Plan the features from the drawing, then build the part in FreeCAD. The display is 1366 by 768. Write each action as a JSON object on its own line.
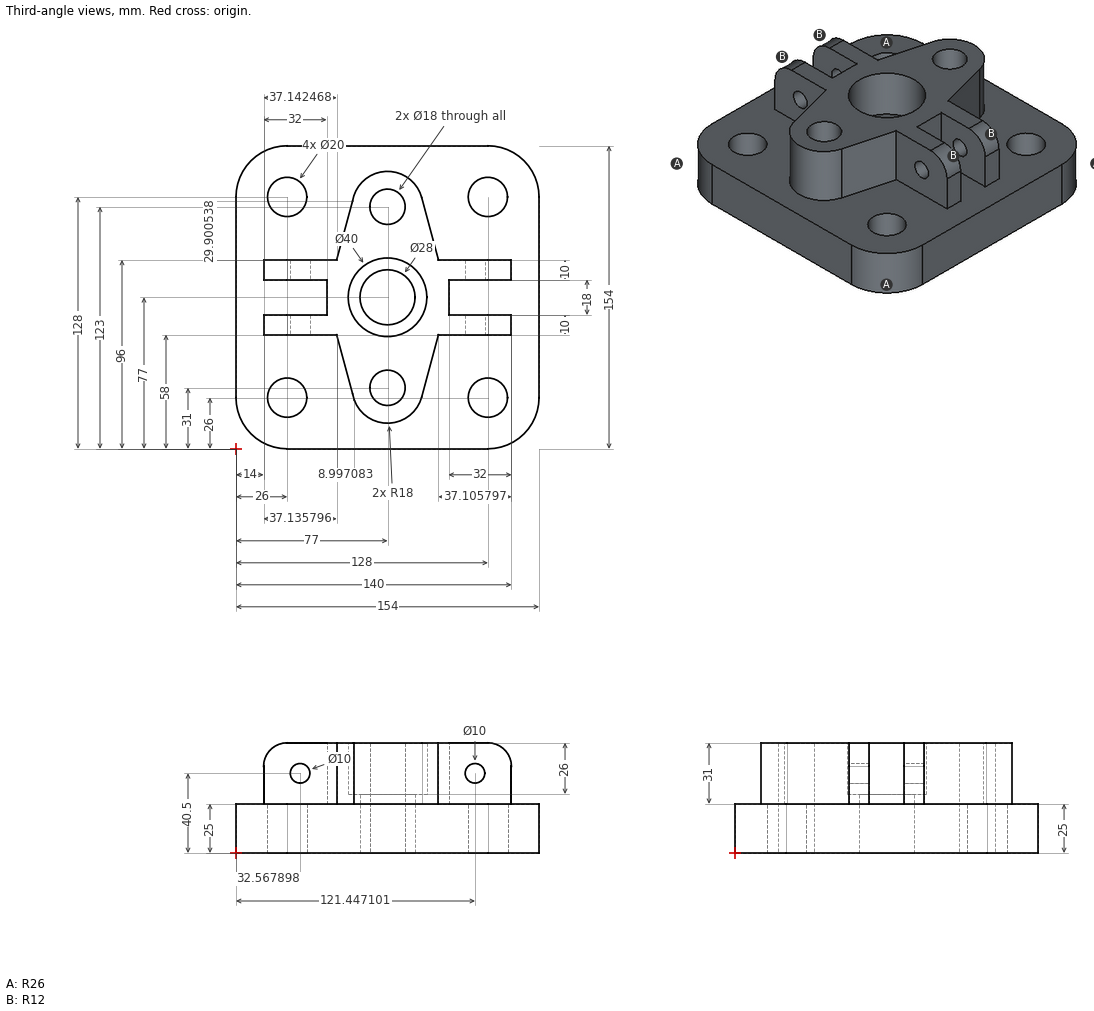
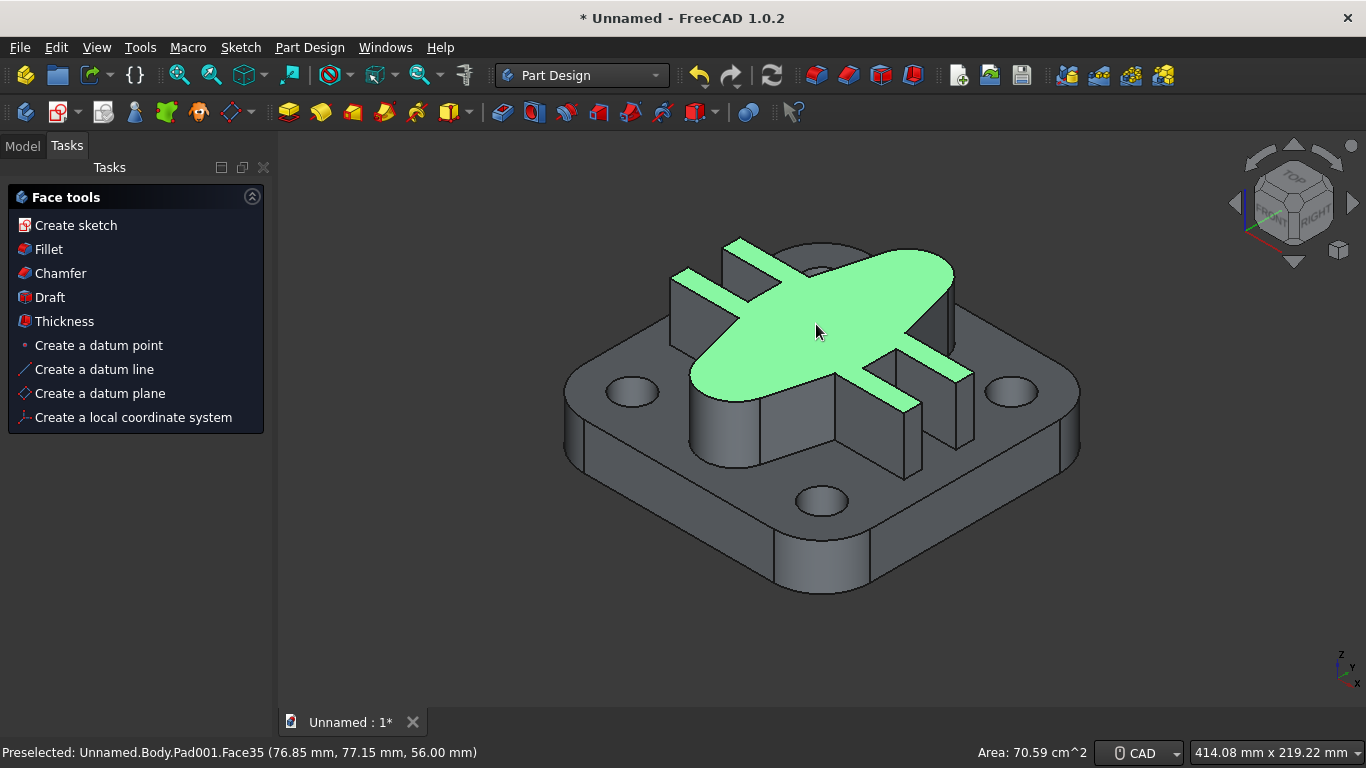
{"action": "left_click", "coordinate": [58, 112]}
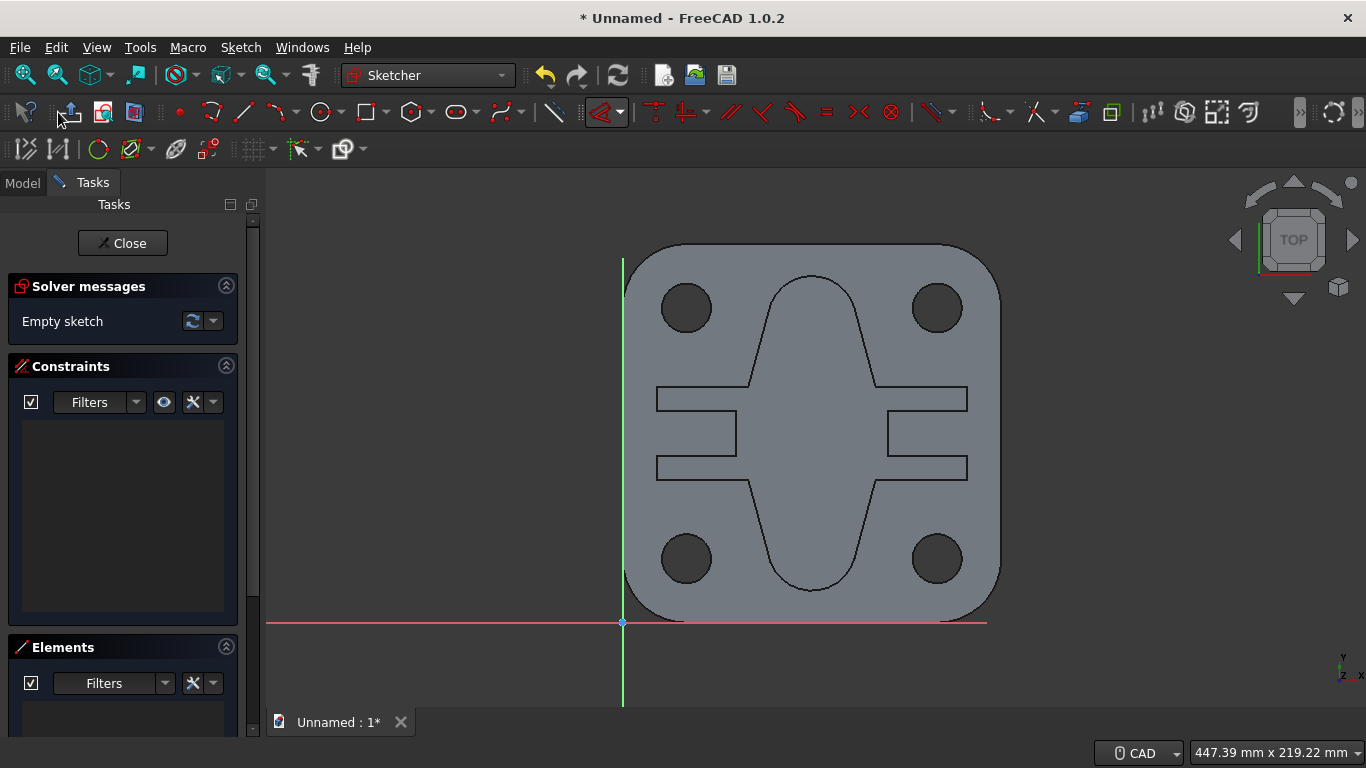
{"action": "left_click", "coordinate": [322, 112]}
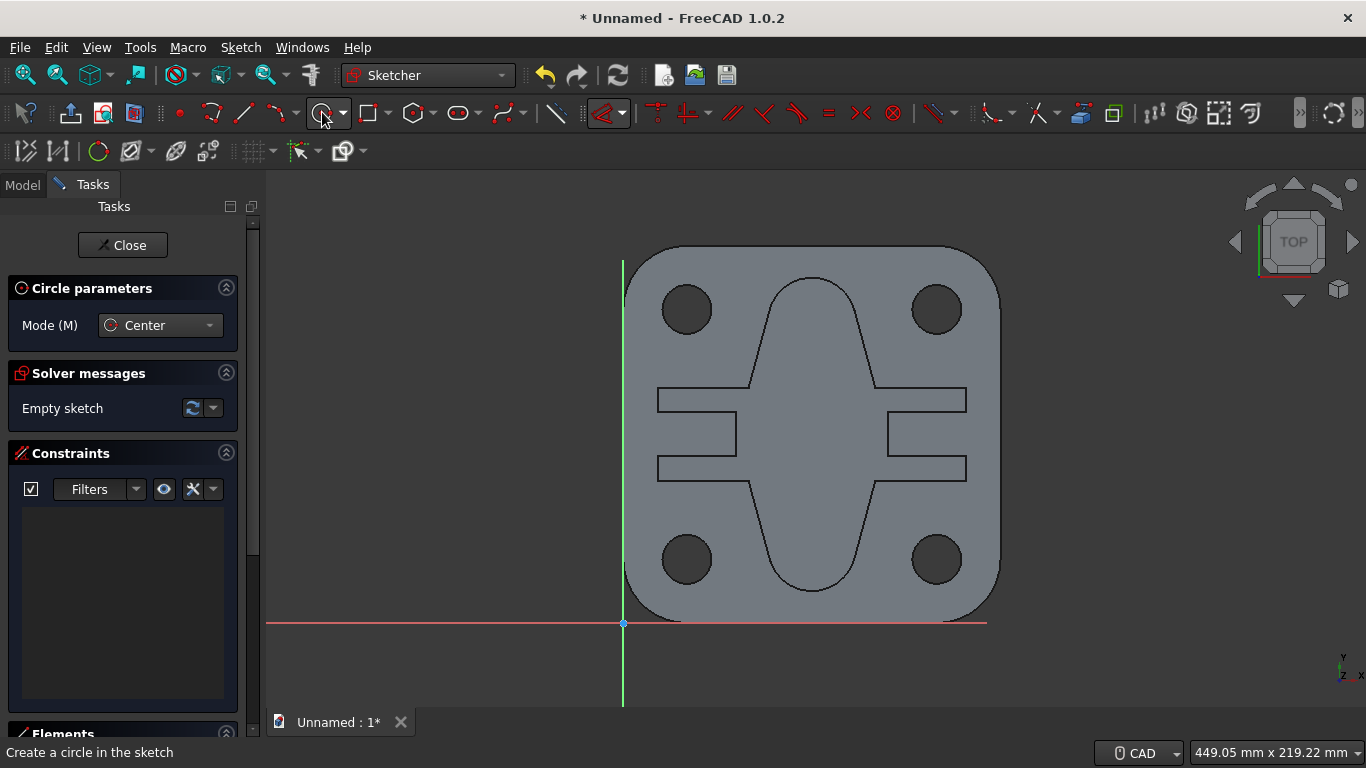
{"action": "left_click", "coordinate": [812, 322]}
{"action": "left_click", "coordinate": [827, 306]}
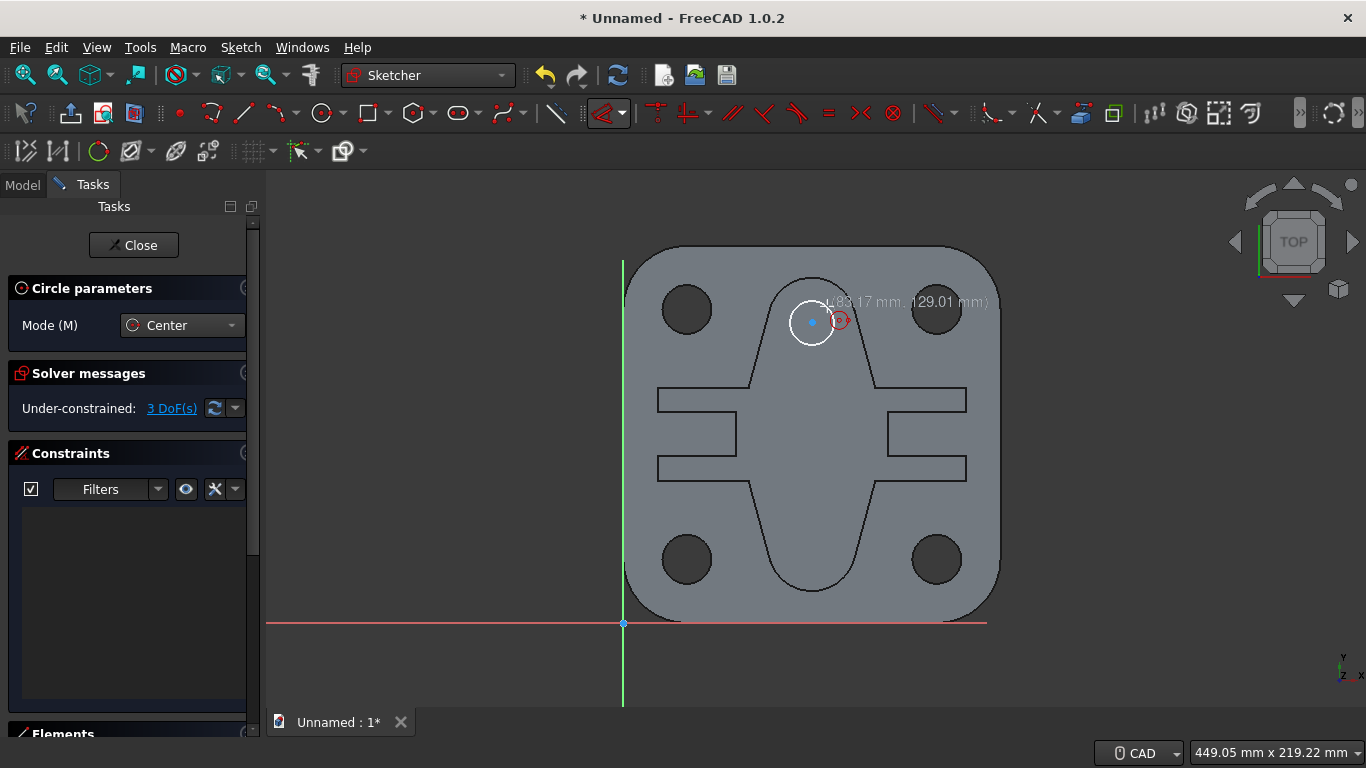
{"action": "left_click", "coordinate": [812, 547]}
{"action": "left_click", "coordinate": [827, 531]}
{"action": "key", "text": "Escape"}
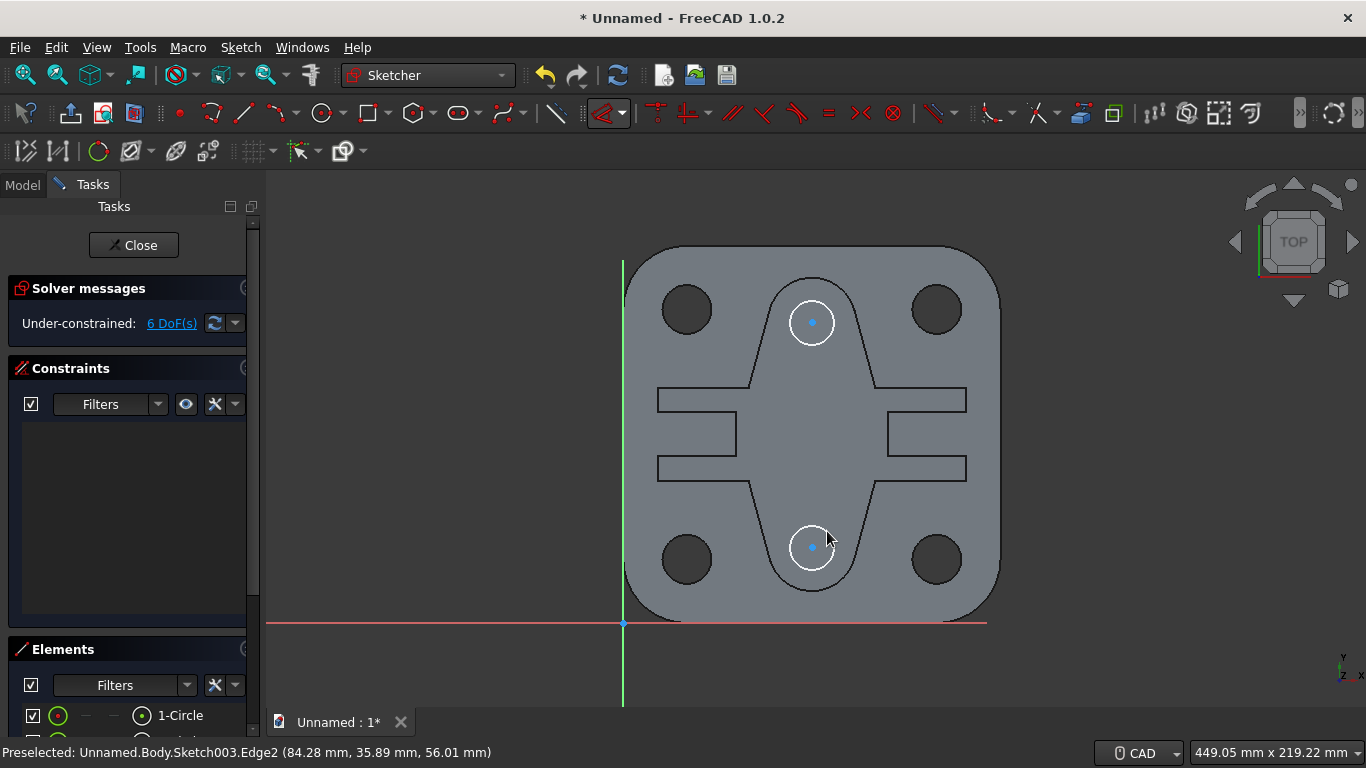
{"action": "left_click", "coordinate": [827, 307]}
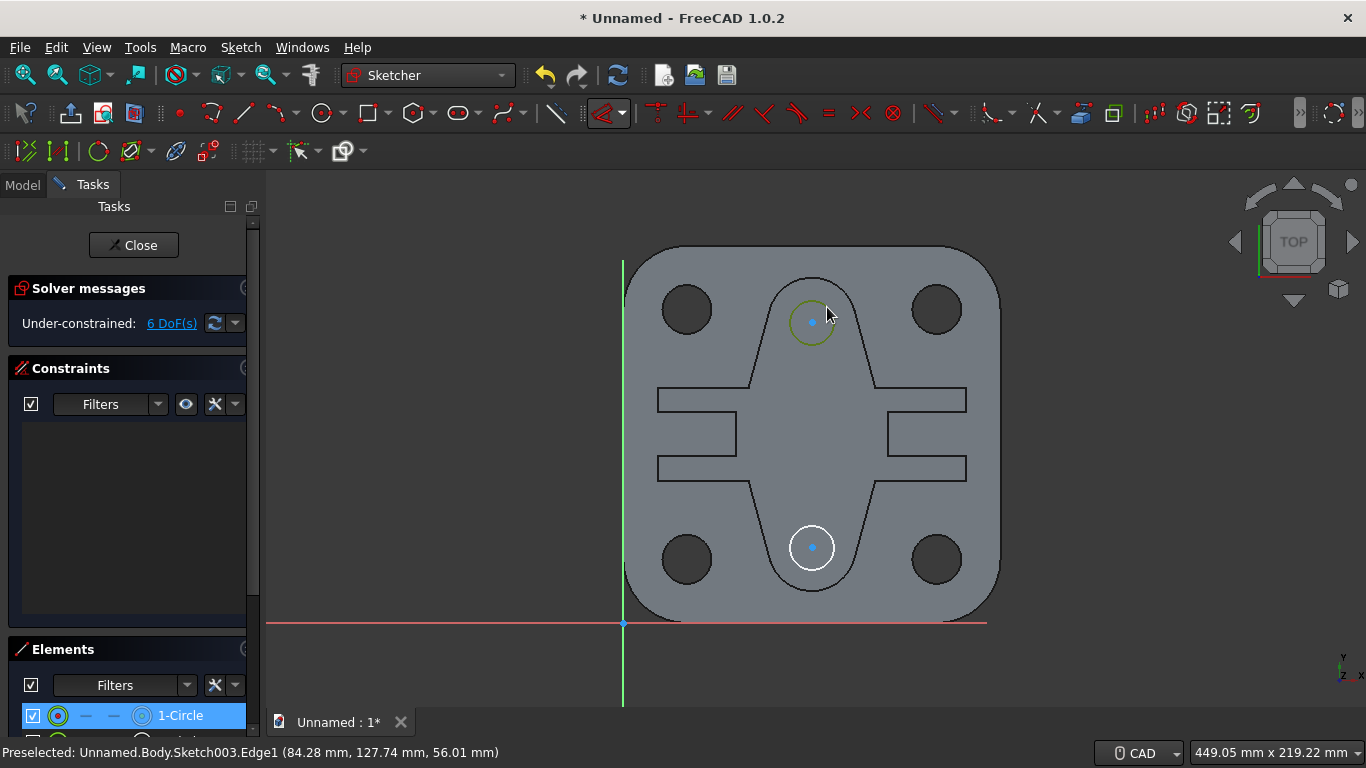
{"action": "left_click", "coordinate": [827, 532]}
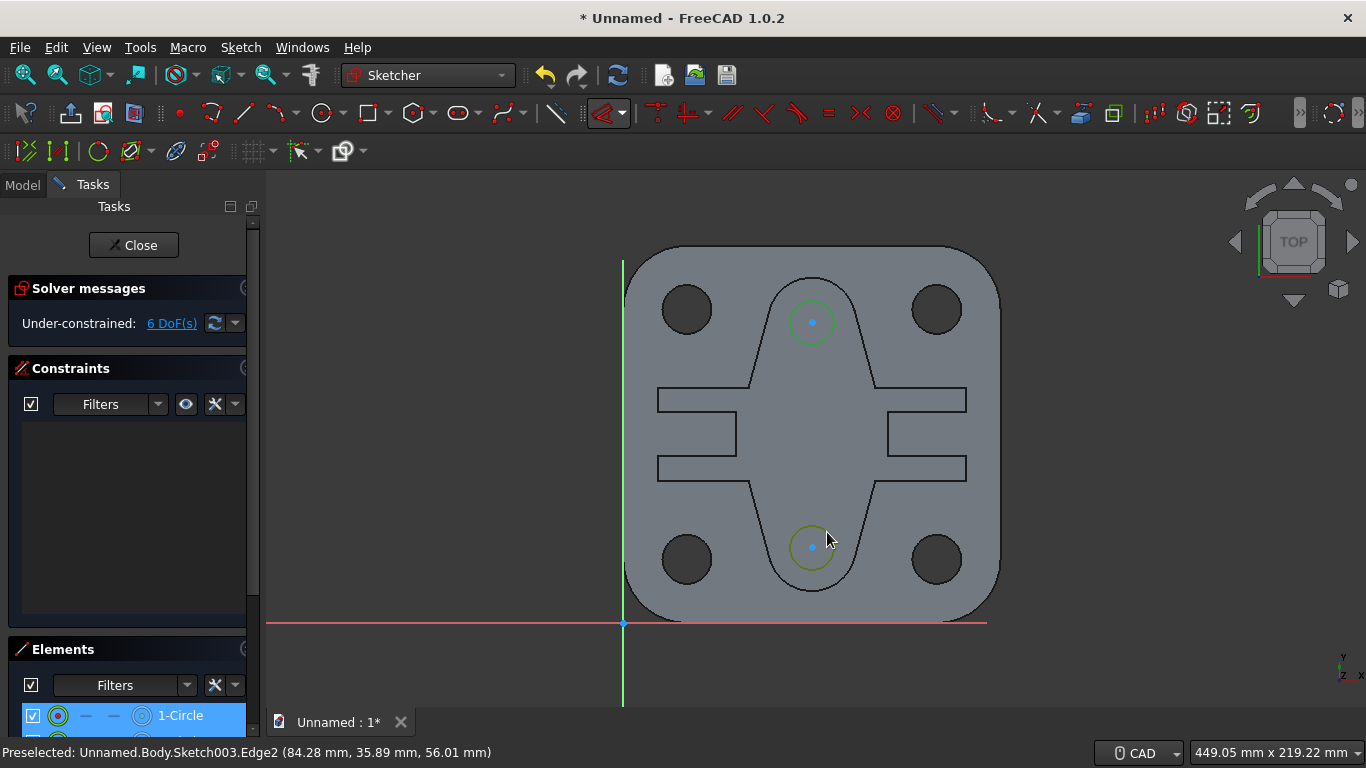
{"action": "left_click", "coordinate": [830, 114]}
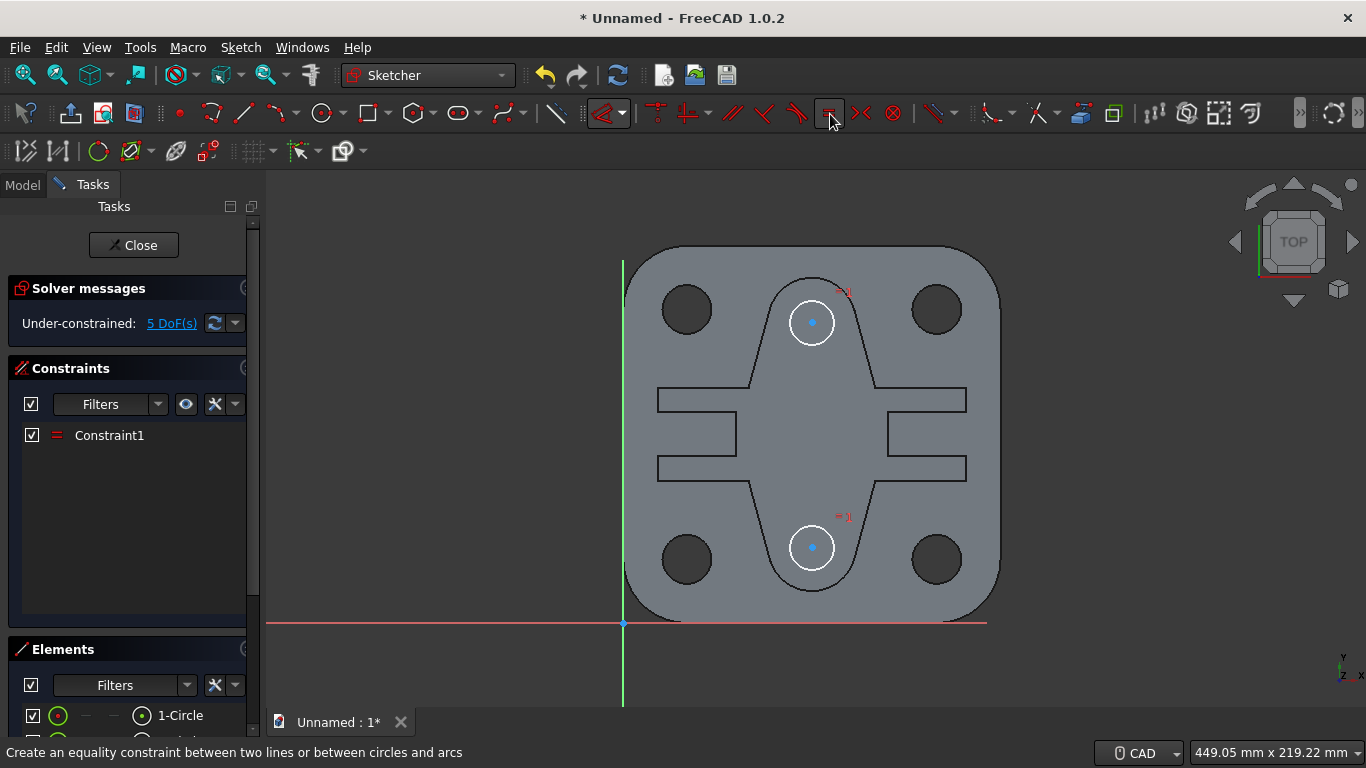
{"action": "left_click", "coordinate": [827, 307]}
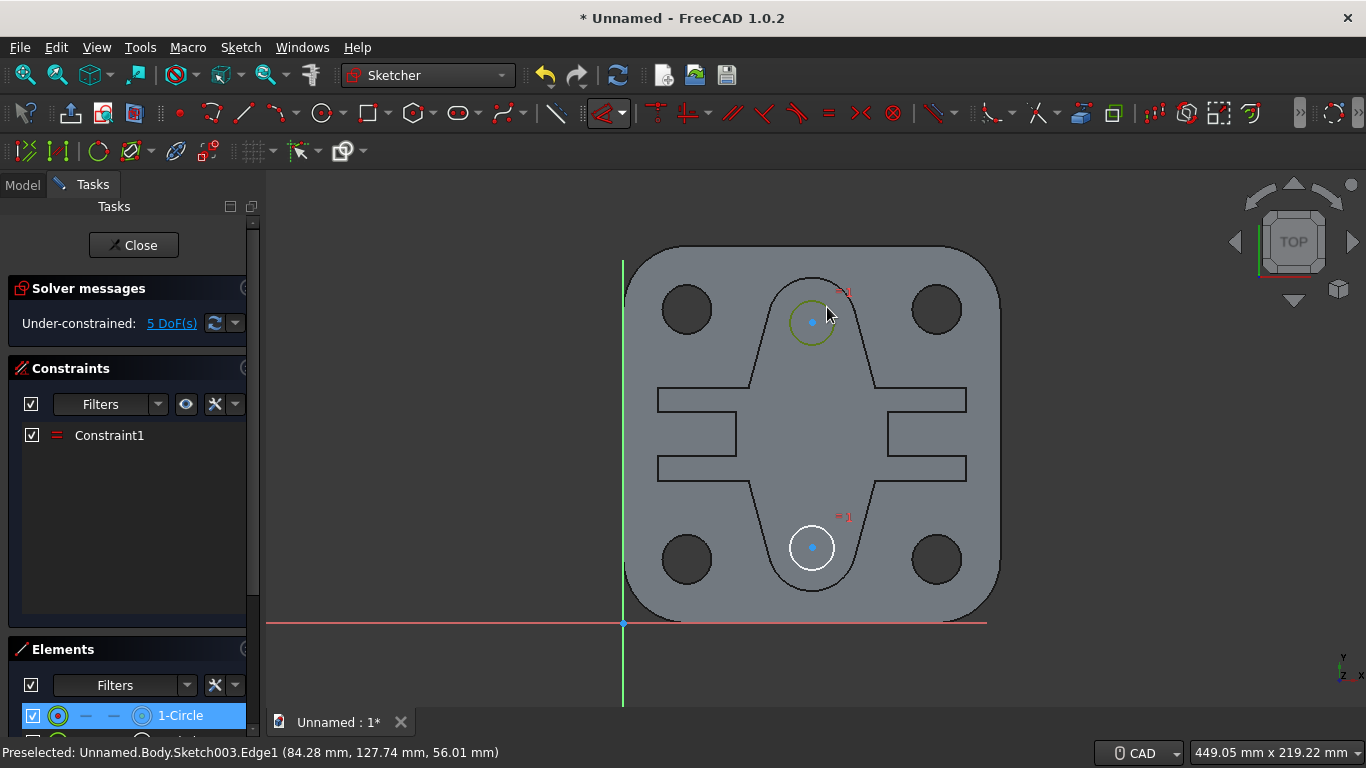
{"action": "key", "text": "k o"}